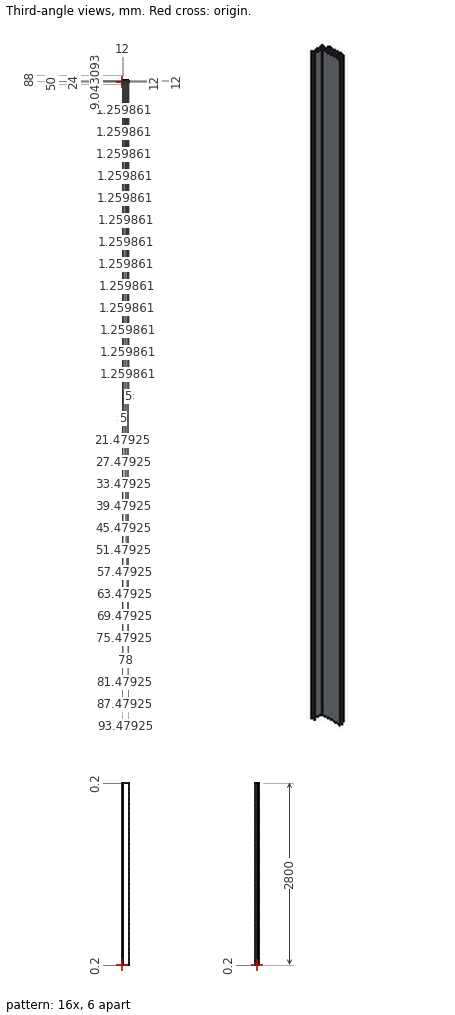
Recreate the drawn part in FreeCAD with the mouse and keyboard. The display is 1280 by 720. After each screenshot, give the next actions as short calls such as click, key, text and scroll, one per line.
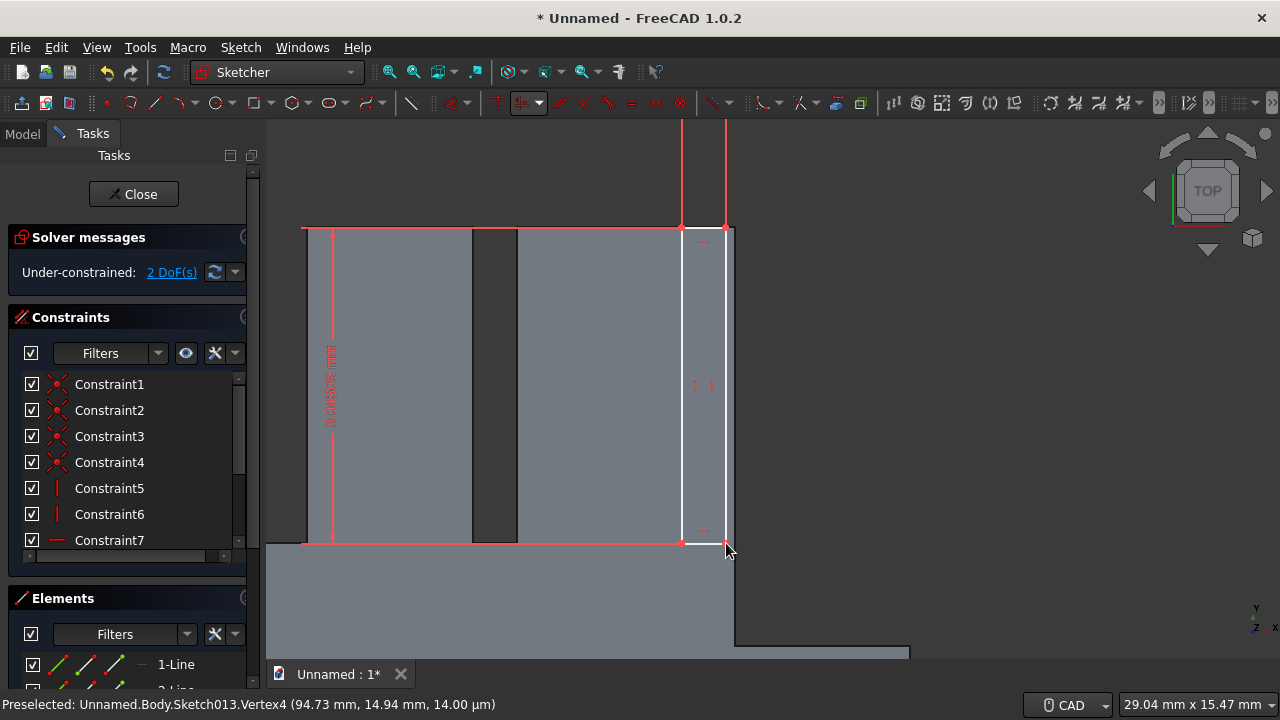
click(450, 104)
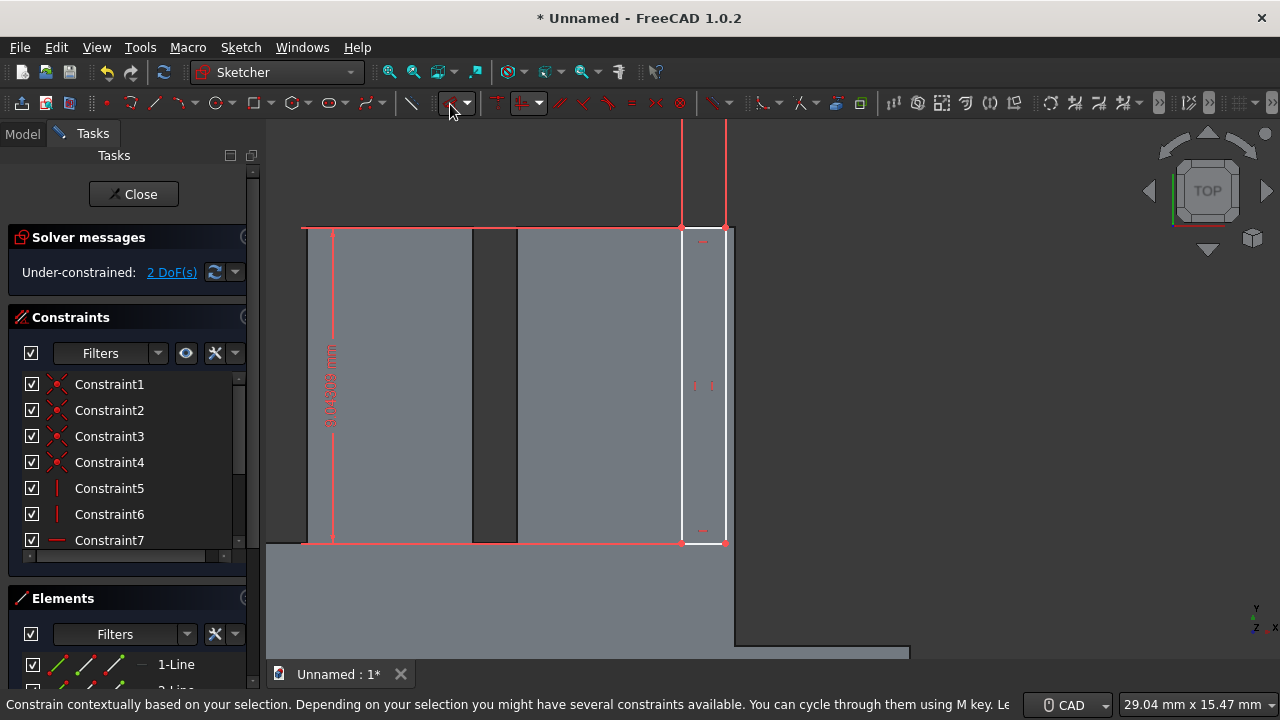
click(682, 228)
click(716, 571)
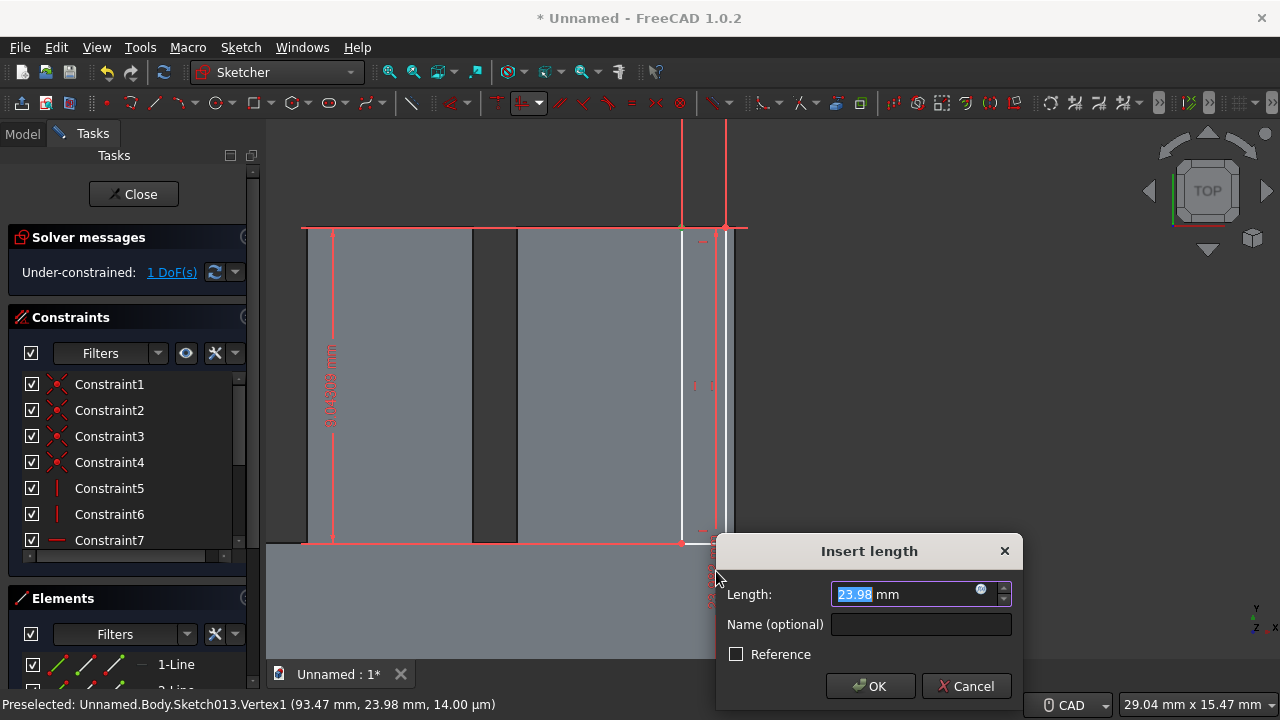
text(24)
key(Return)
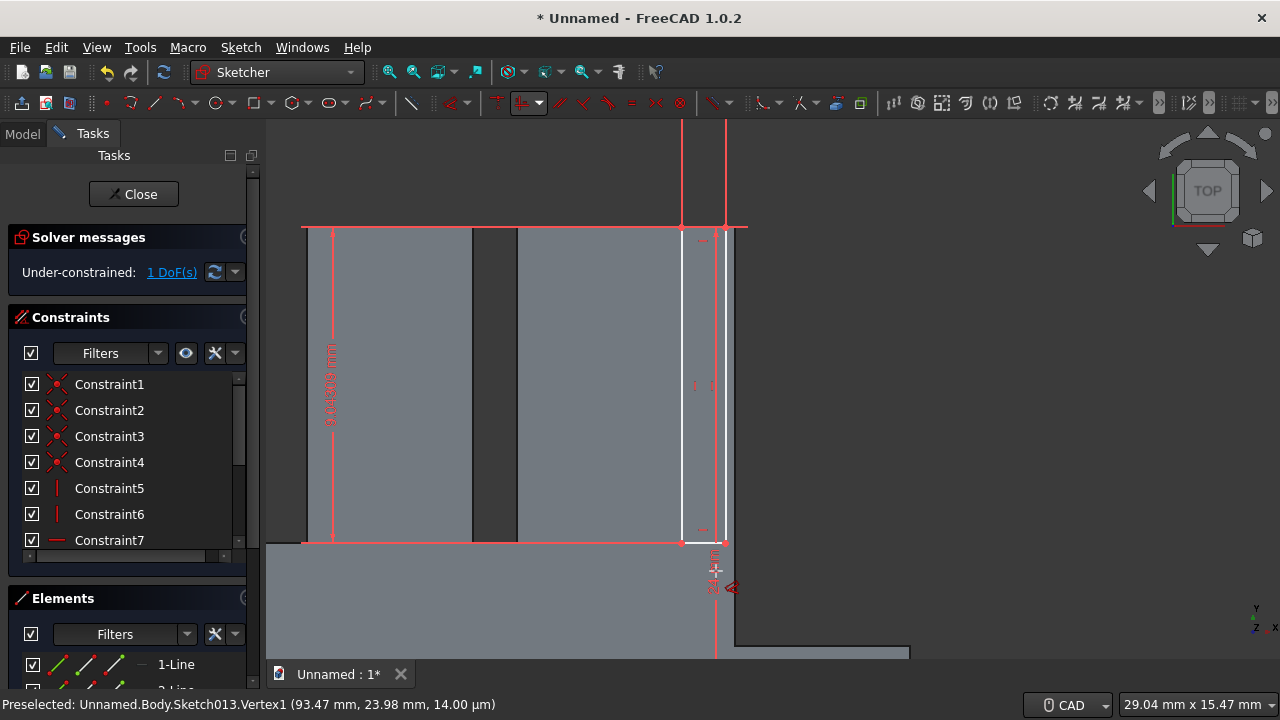
click(682, 227)
click(488, 193)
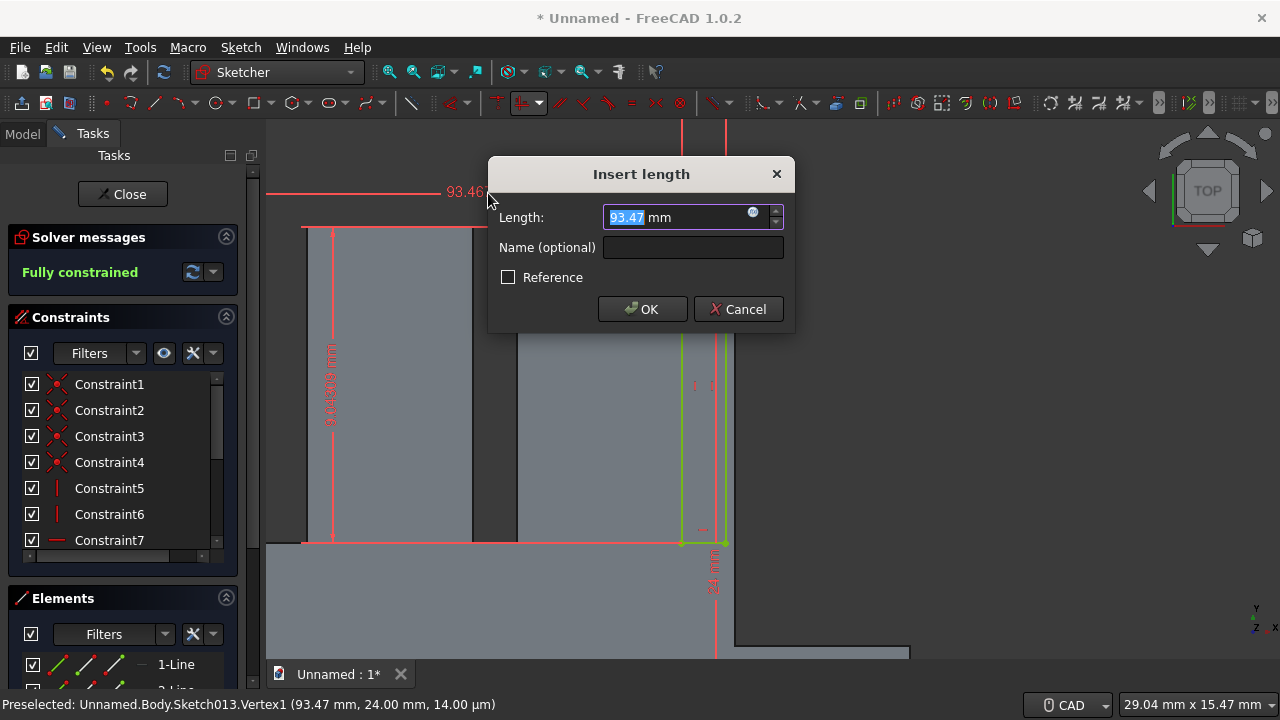
text(93.47925)
key(Return)
key(Escape)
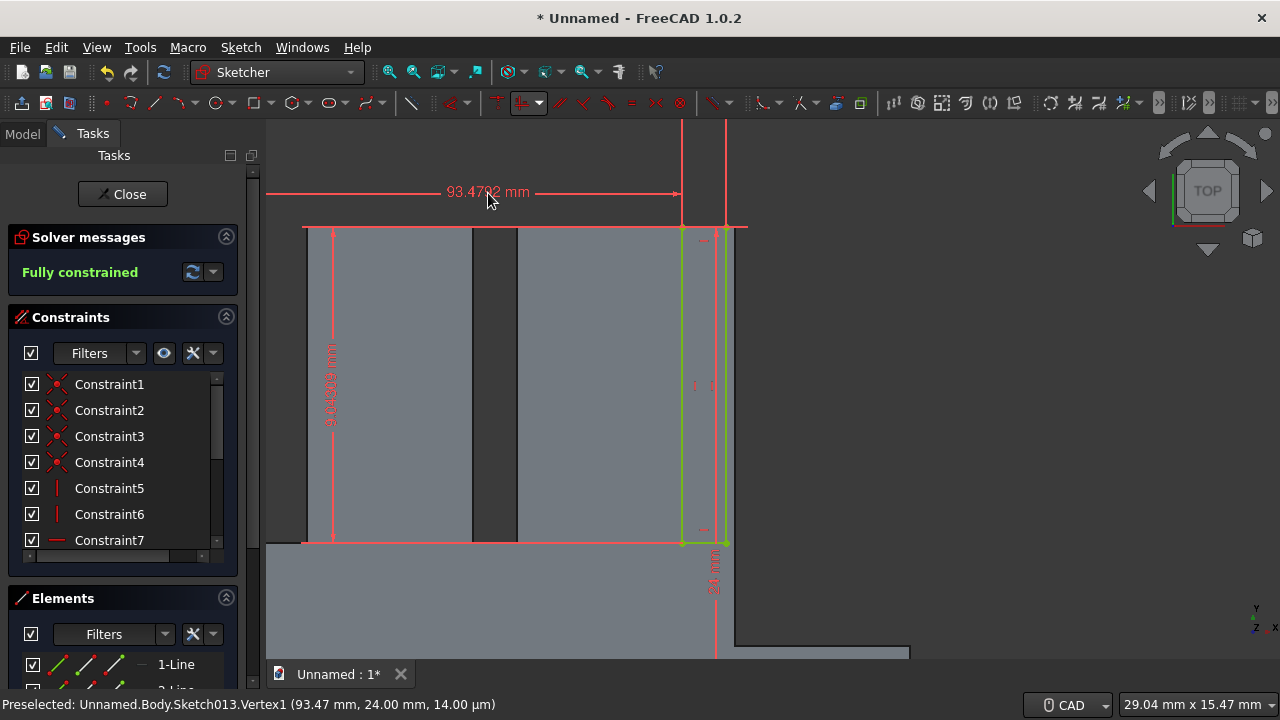
click(123, 194)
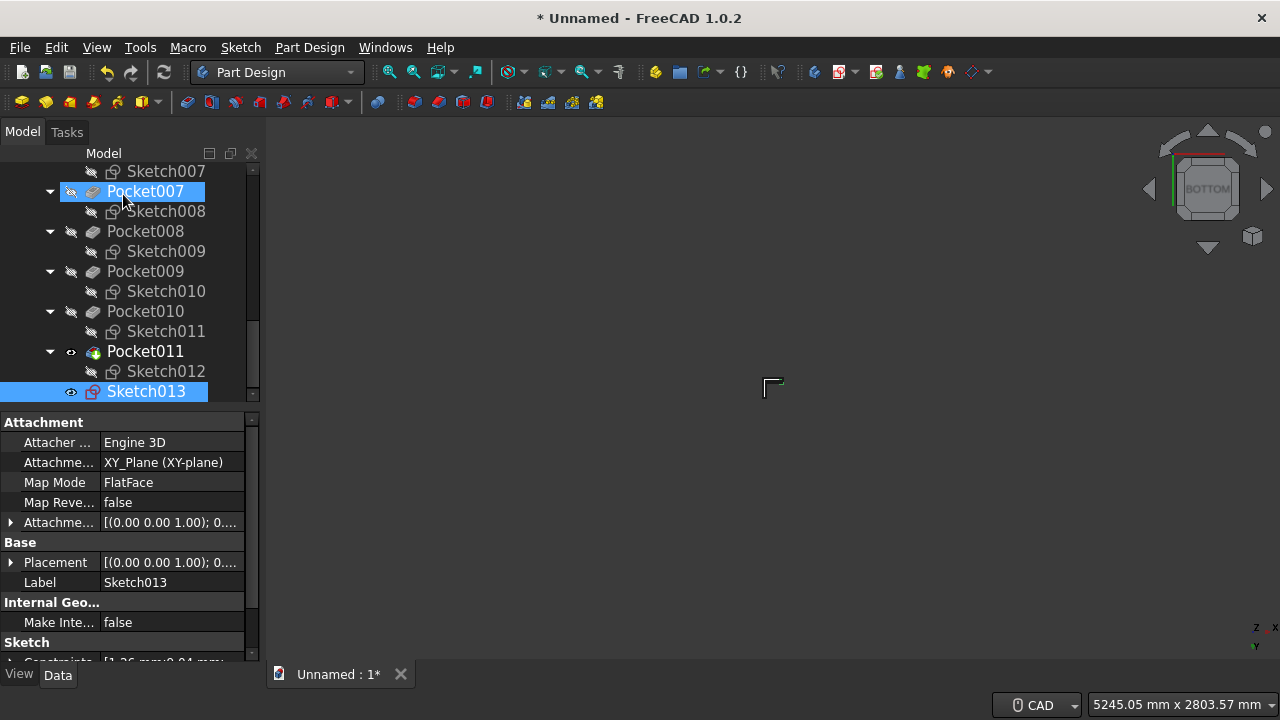
click(188, 102)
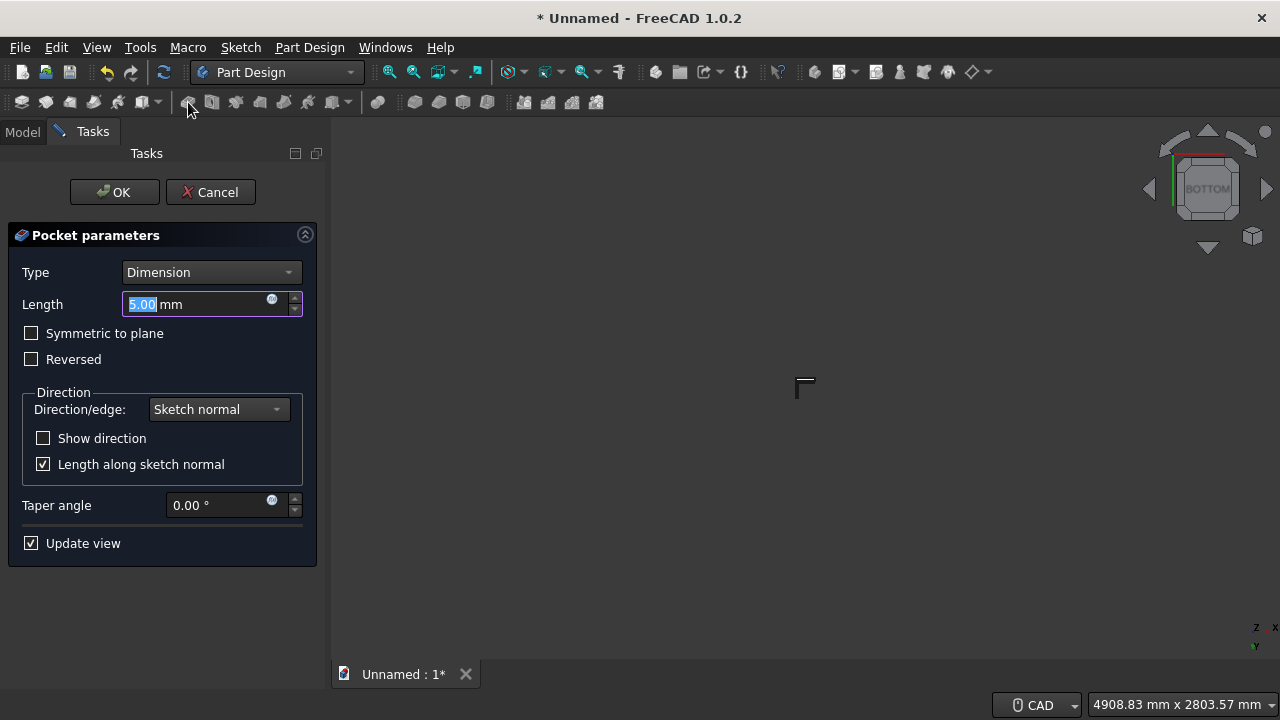
text(0.2)
key(Tab)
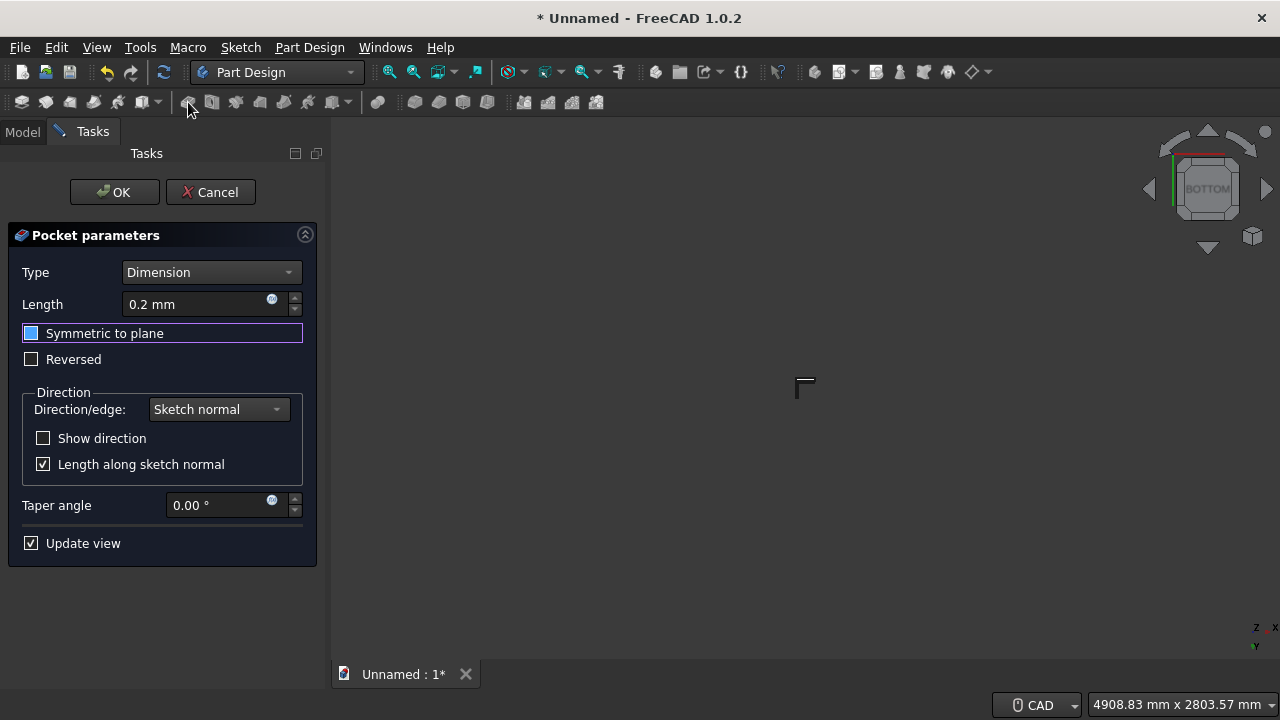
click(30, 359)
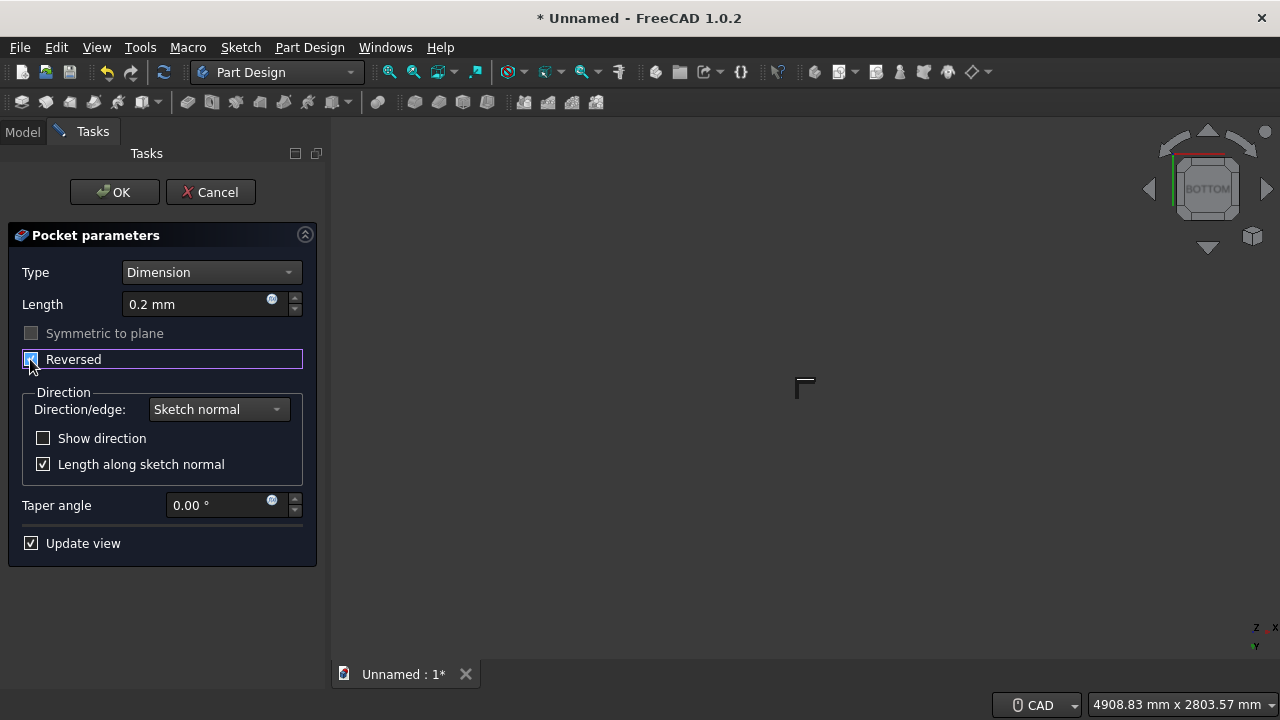
click(115, 192)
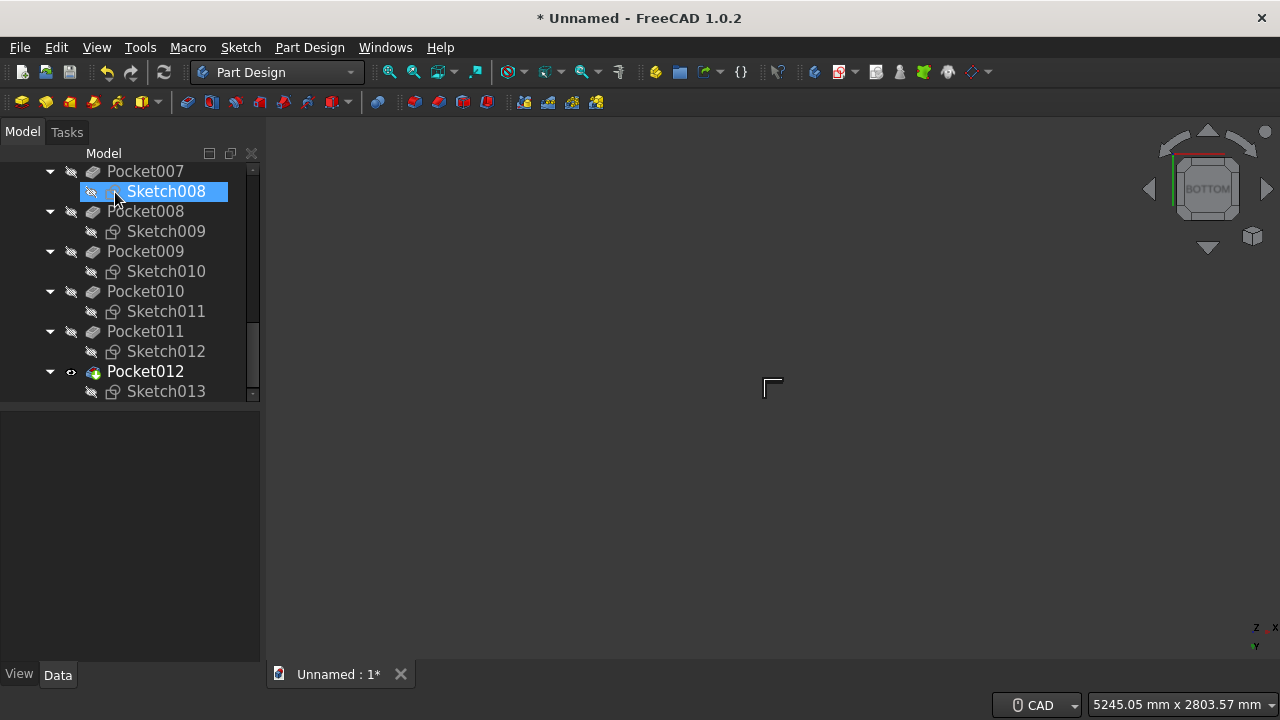
click(390, 72)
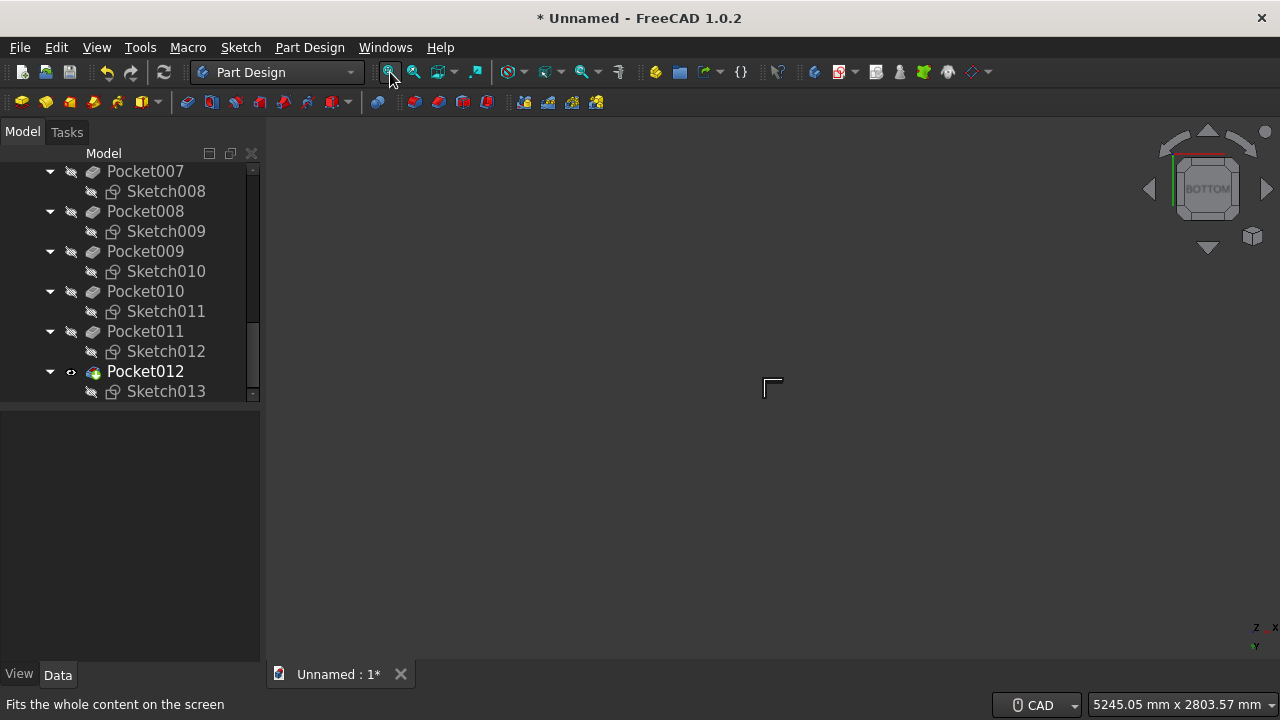
key(0)